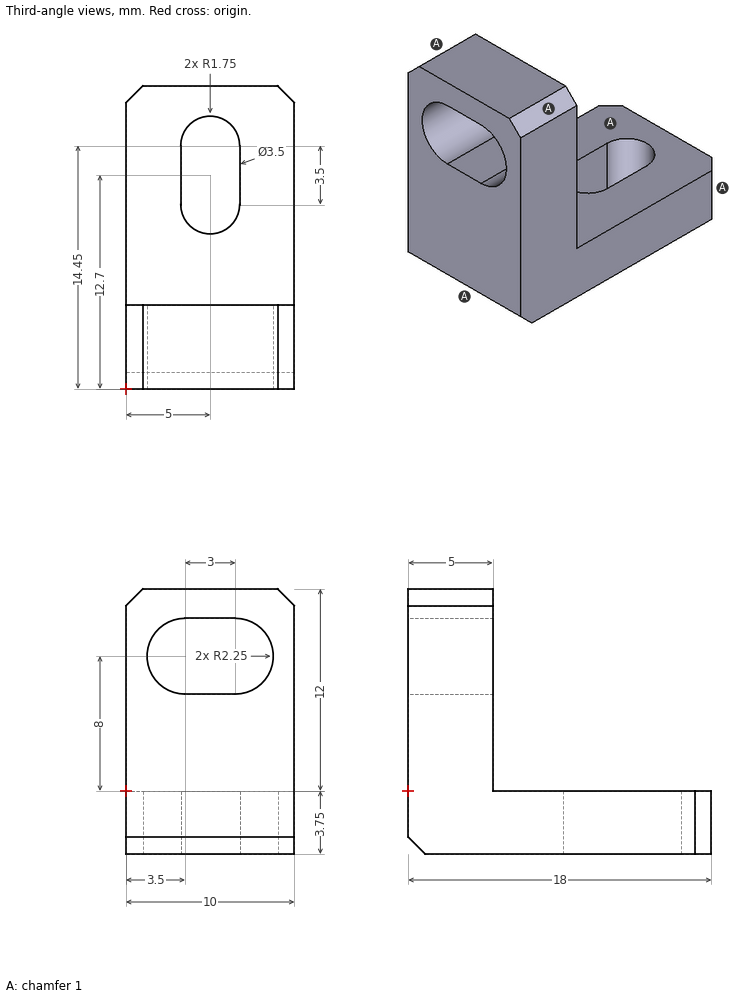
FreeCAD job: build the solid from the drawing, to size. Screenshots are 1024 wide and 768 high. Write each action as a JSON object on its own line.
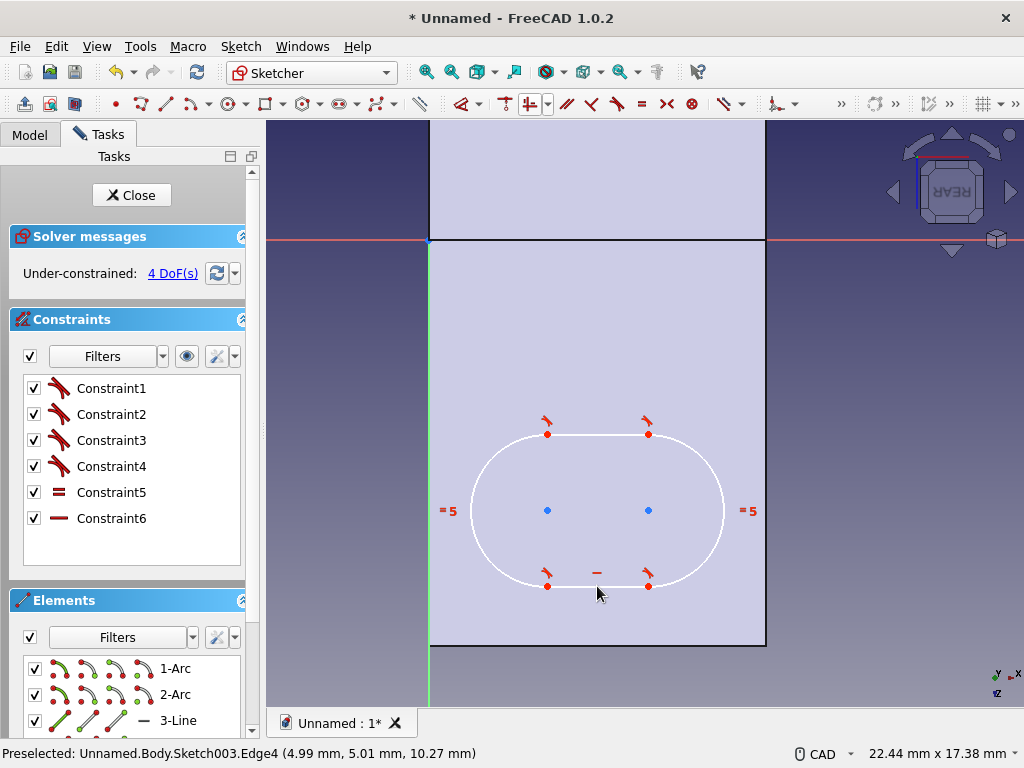
{"action": "left_click", "coordinate": [460, 104]}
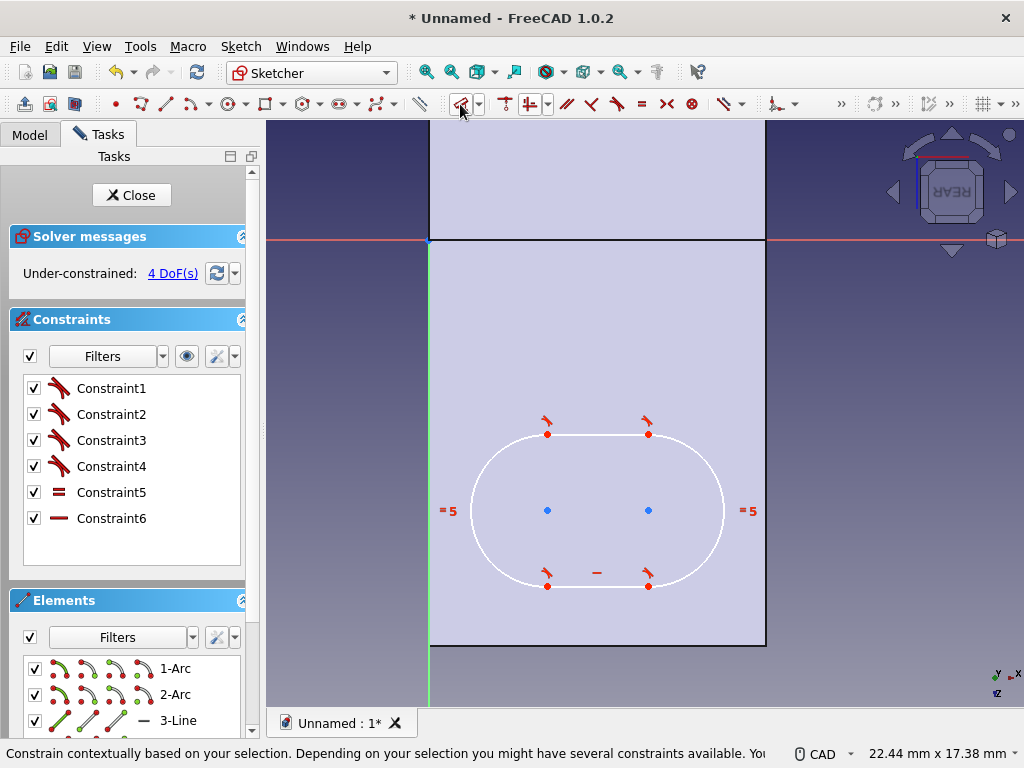
{"action": "left_click", "coordinate": [486, 466]}
{"action": "left_click", "coordinate": [460, 447]}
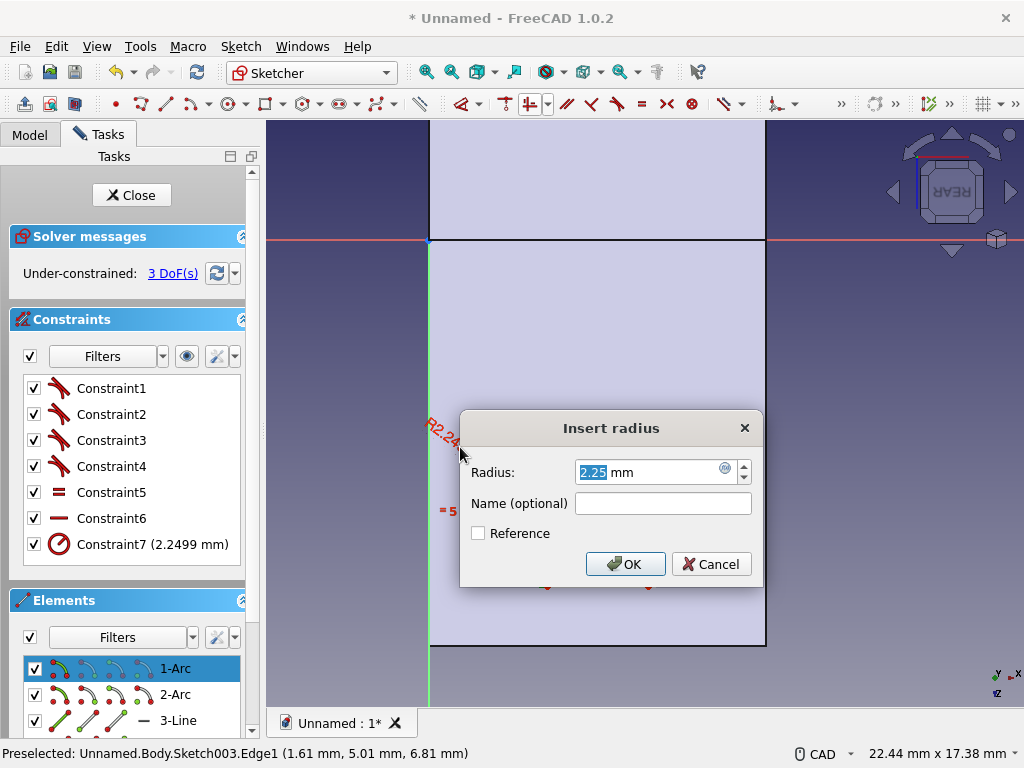
{"action": "type", "text": "2.25"}
{"action": "key", "text": "Return"}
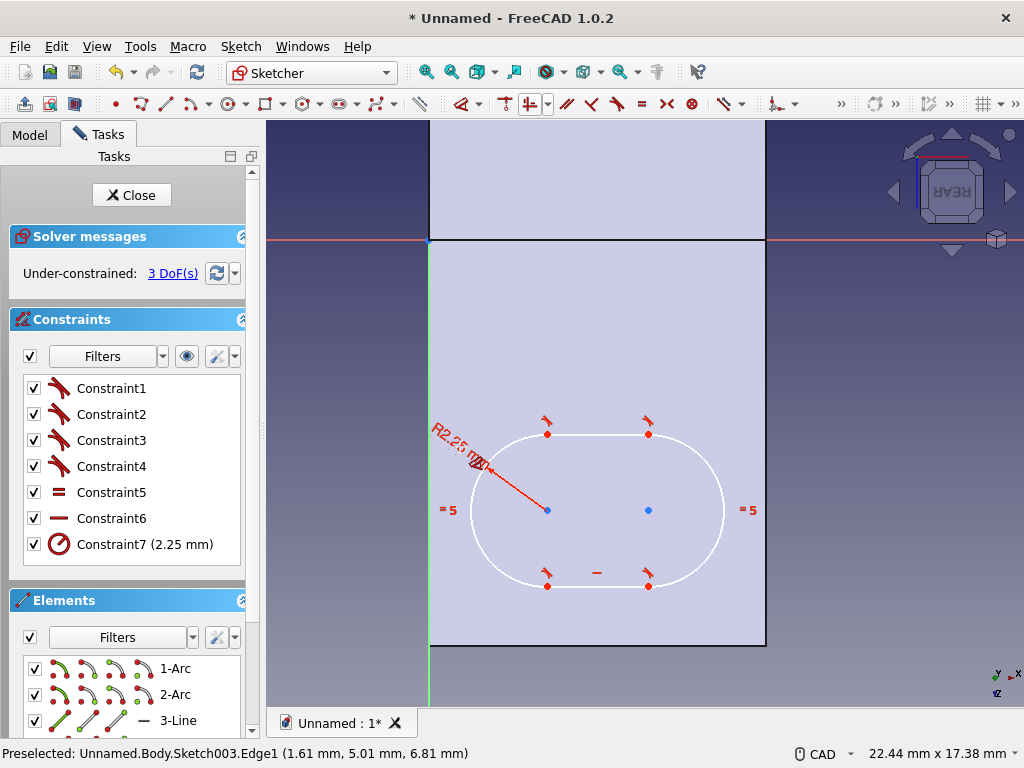
{"action": "left_click", "coordinate": [577, 435]}
{"action": "left_click", "coordinate": [598, 469]}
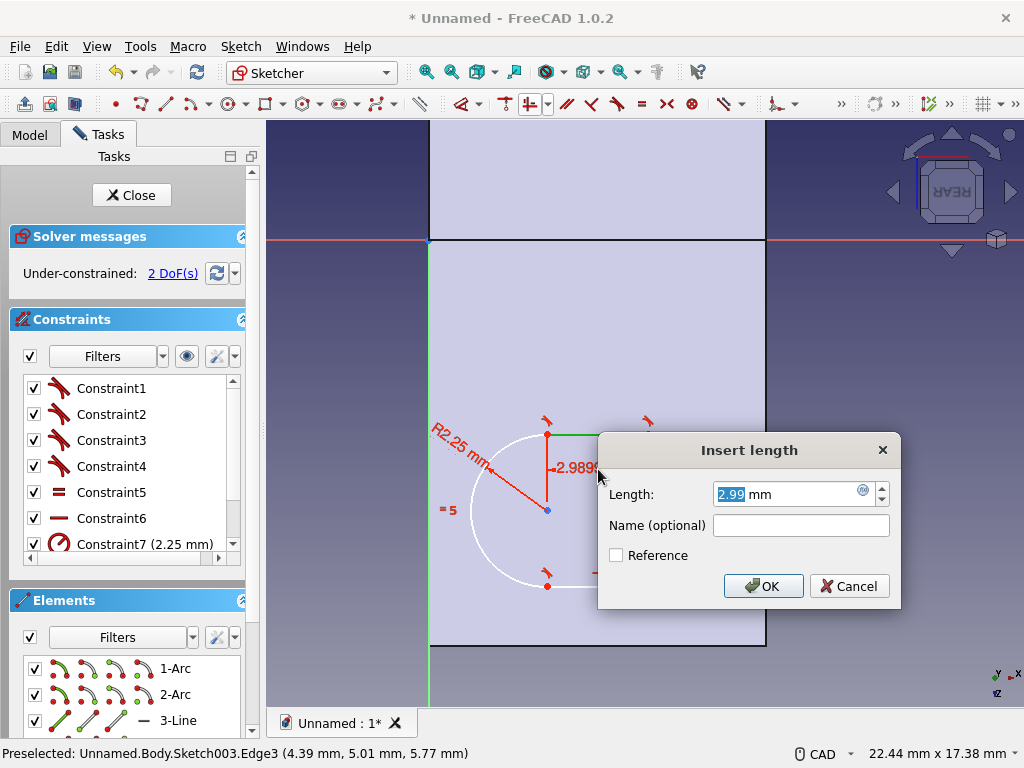
{"action": "type", "text": "3"}
{"action": "key", "text": "Return"}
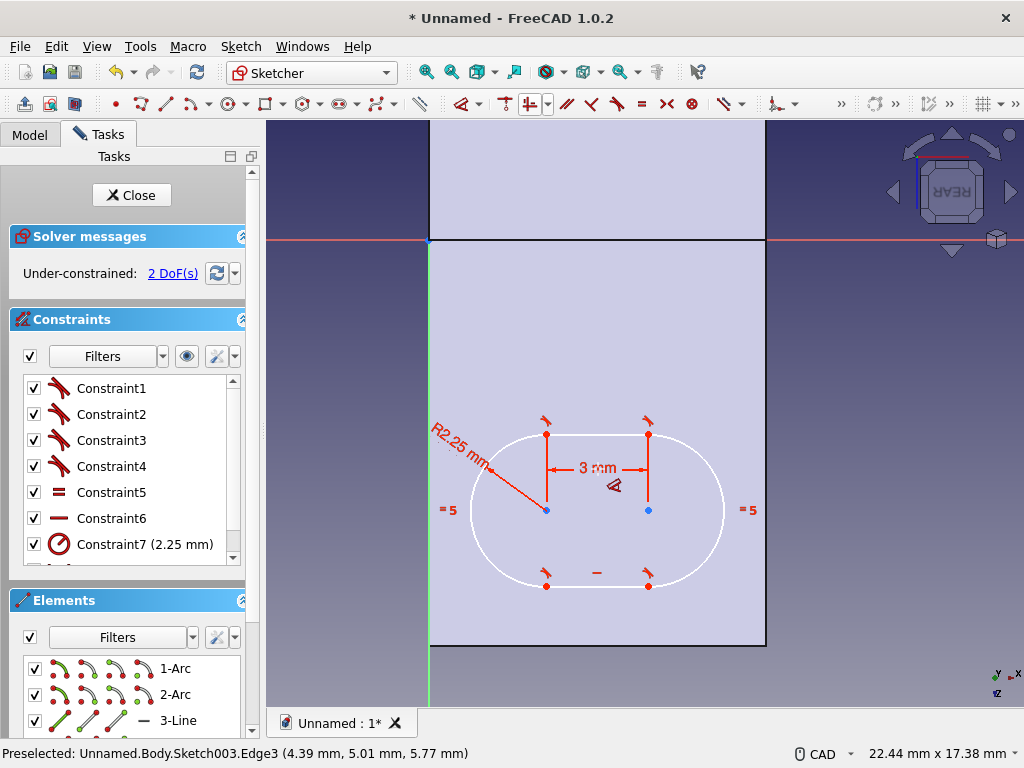
{"action": "left_click", "coordinate": [547, 511]}
{"action": "left_click", "coordinate": [395, 376]}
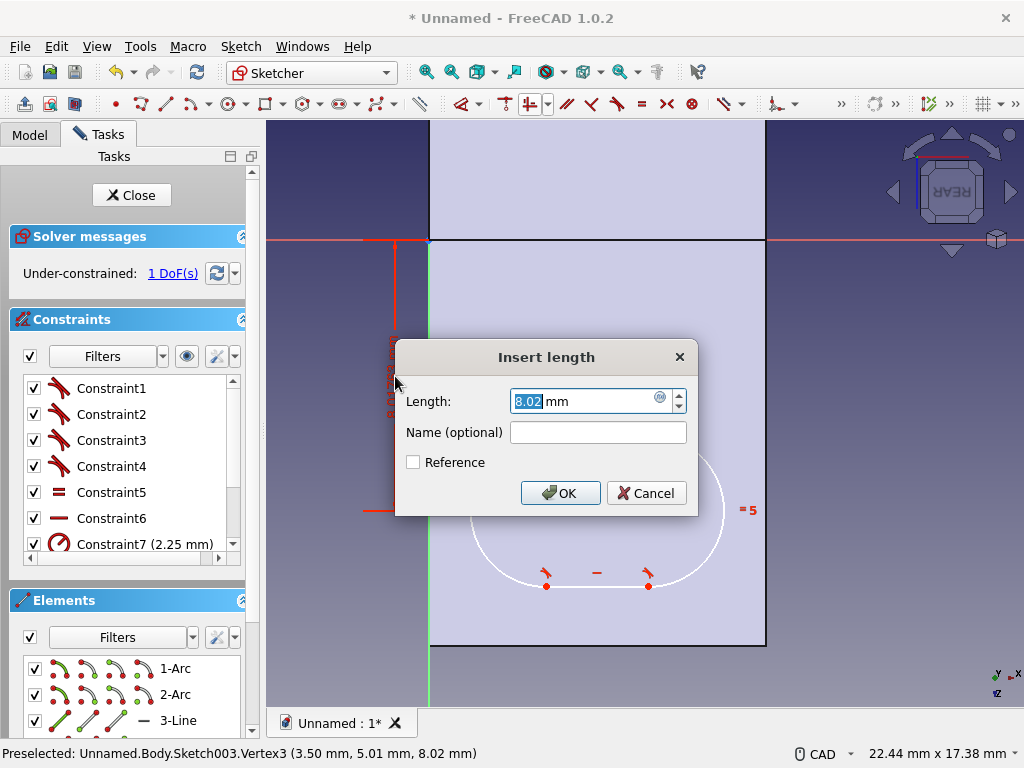
{"action": "type", "text": "8"}
{"action": "key", "text": "Return"}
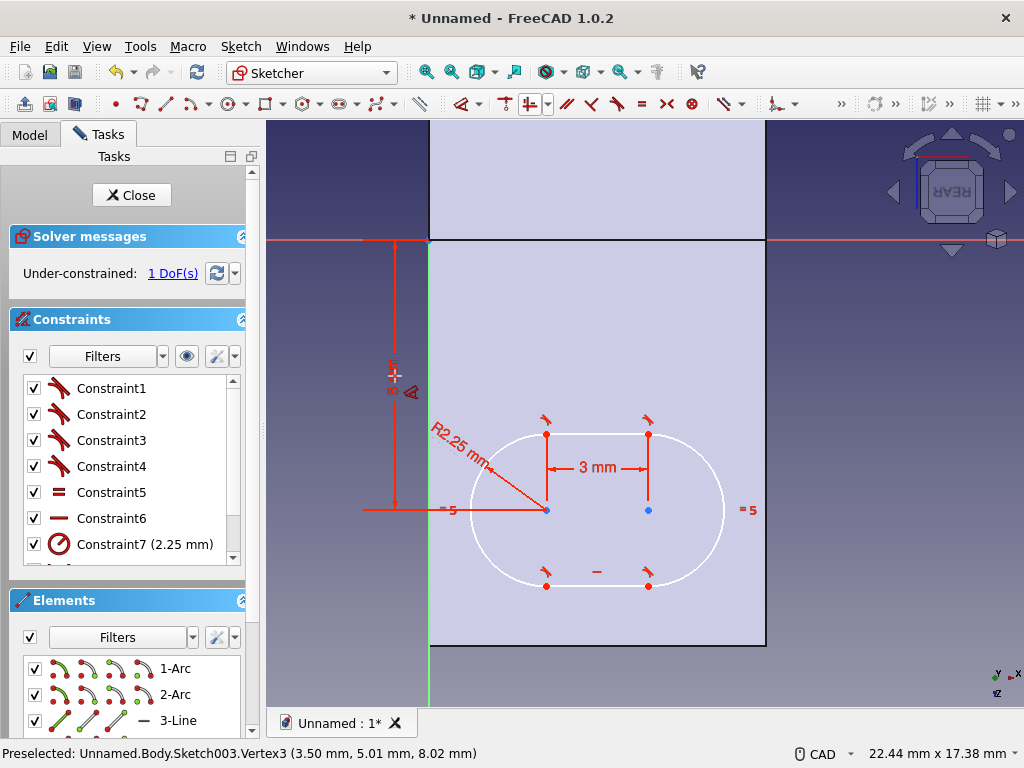
{"action": "left_click", "coordinate": [547, 434]}
{"action": "left_click", "coordinate": [488, 206]}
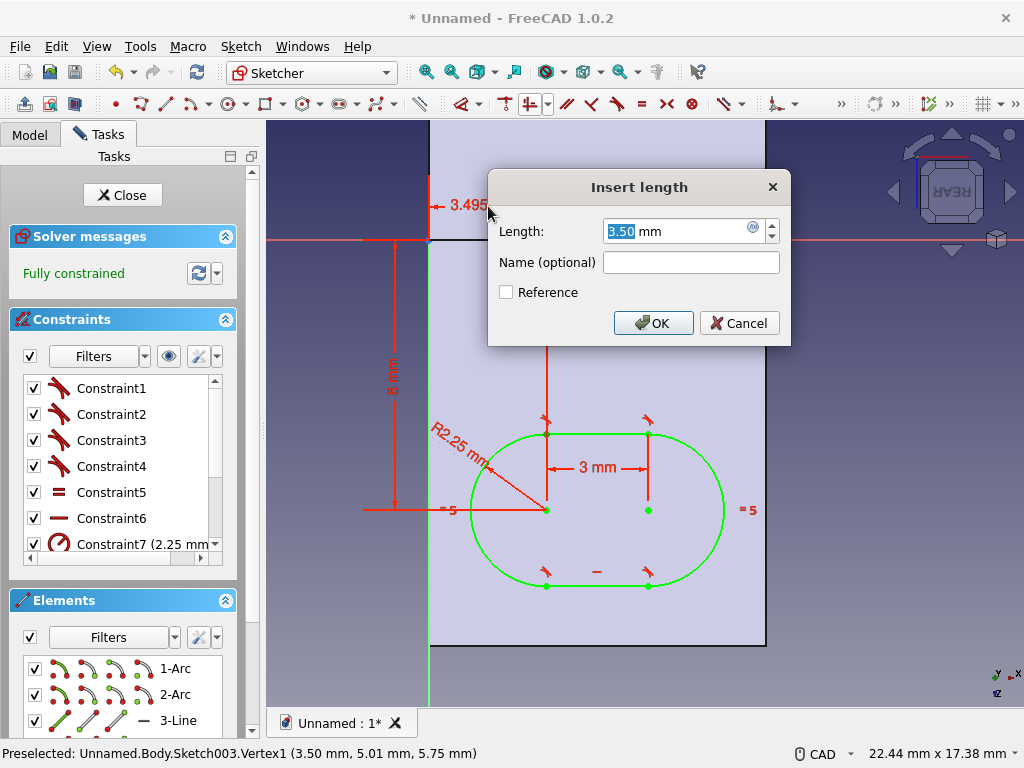
{"action": "type", "text": "3.5"}
{"action": "key", "text": "Return"}
{"action": "key", "text": "Escape"}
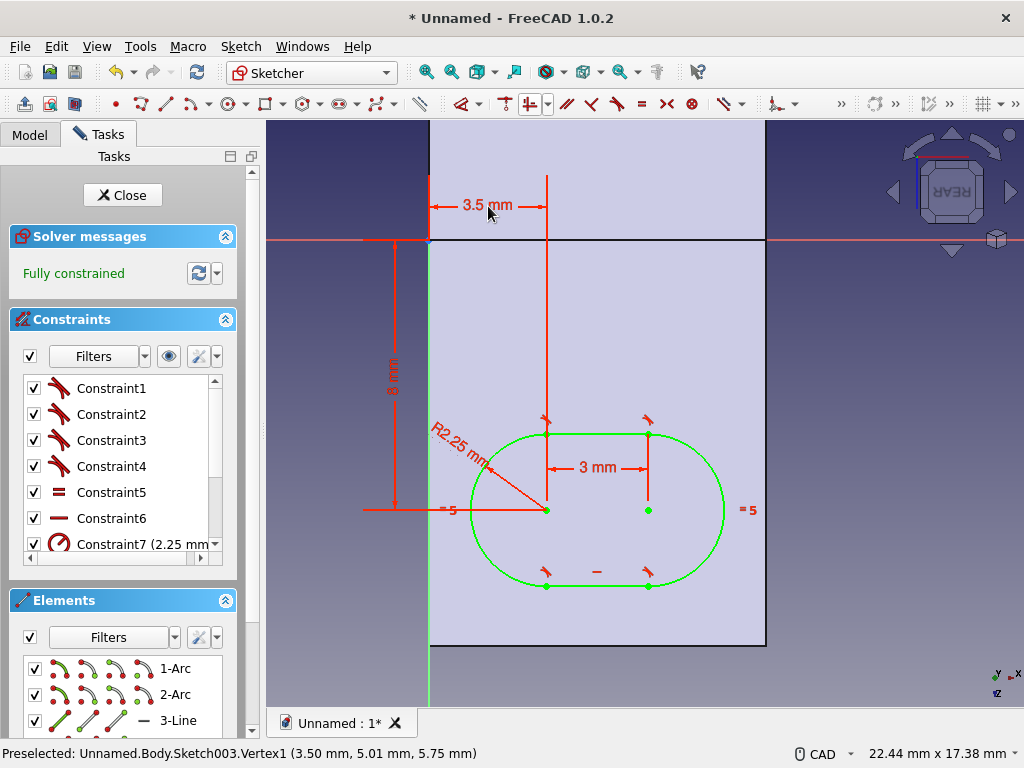
{"action": "left_click", "coordinate": [123, 195]}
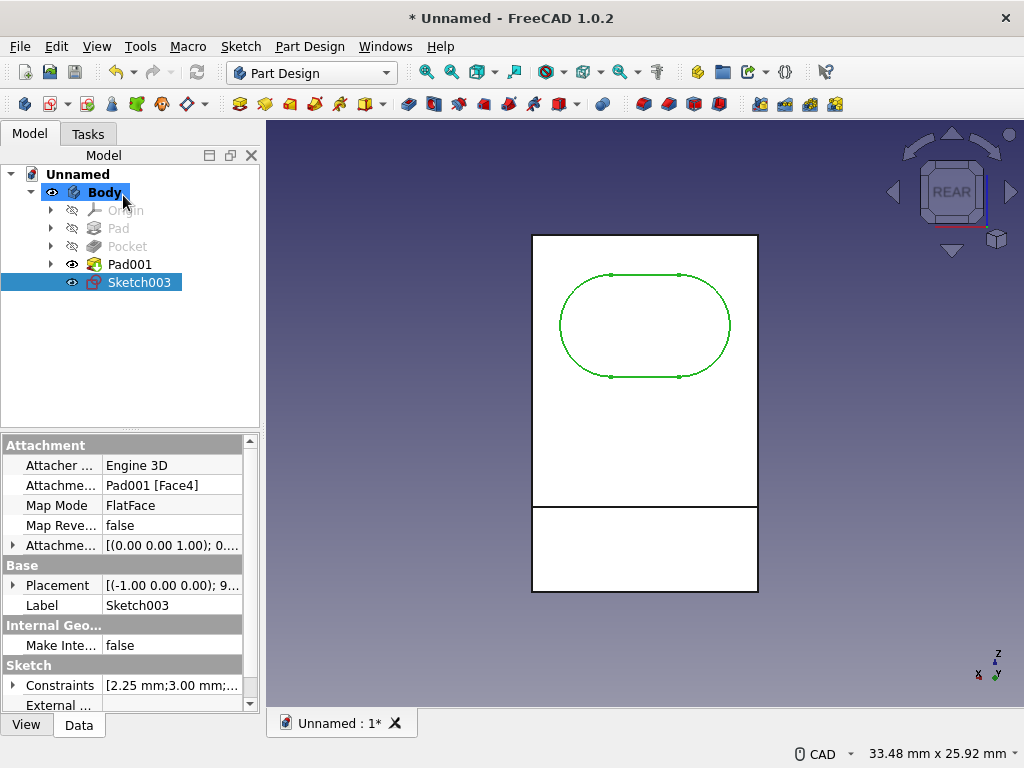
{"action": "left_click", "coordinate": [409, 104]}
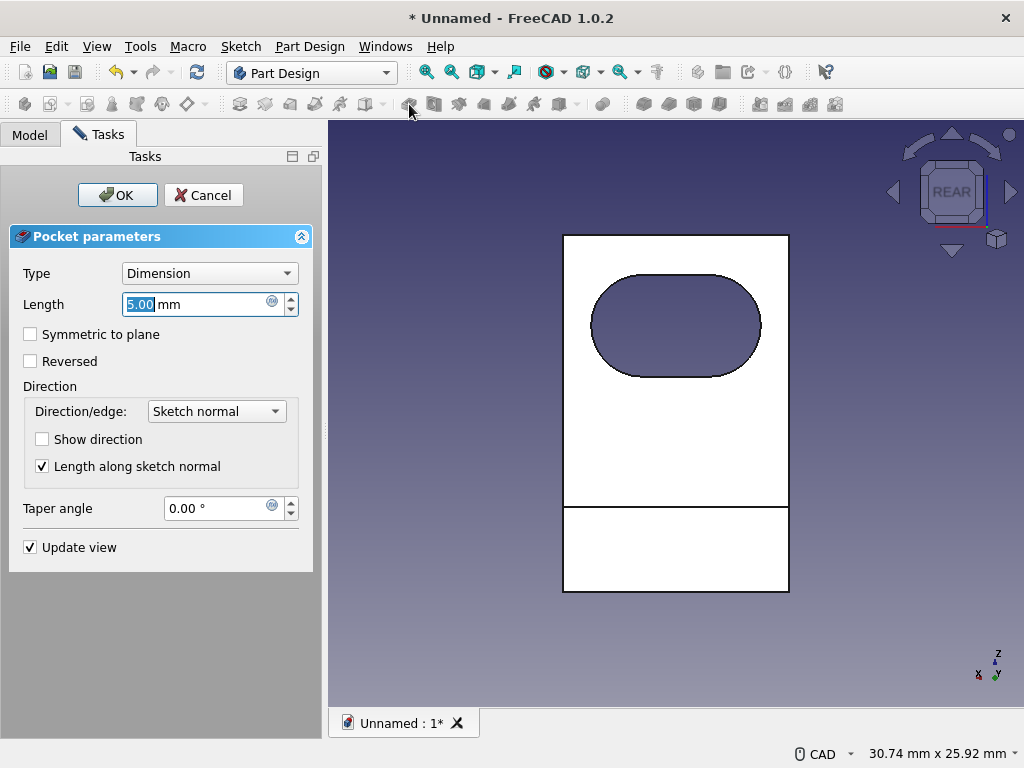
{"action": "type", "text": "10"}
{"action": "key", "text": "Tab"}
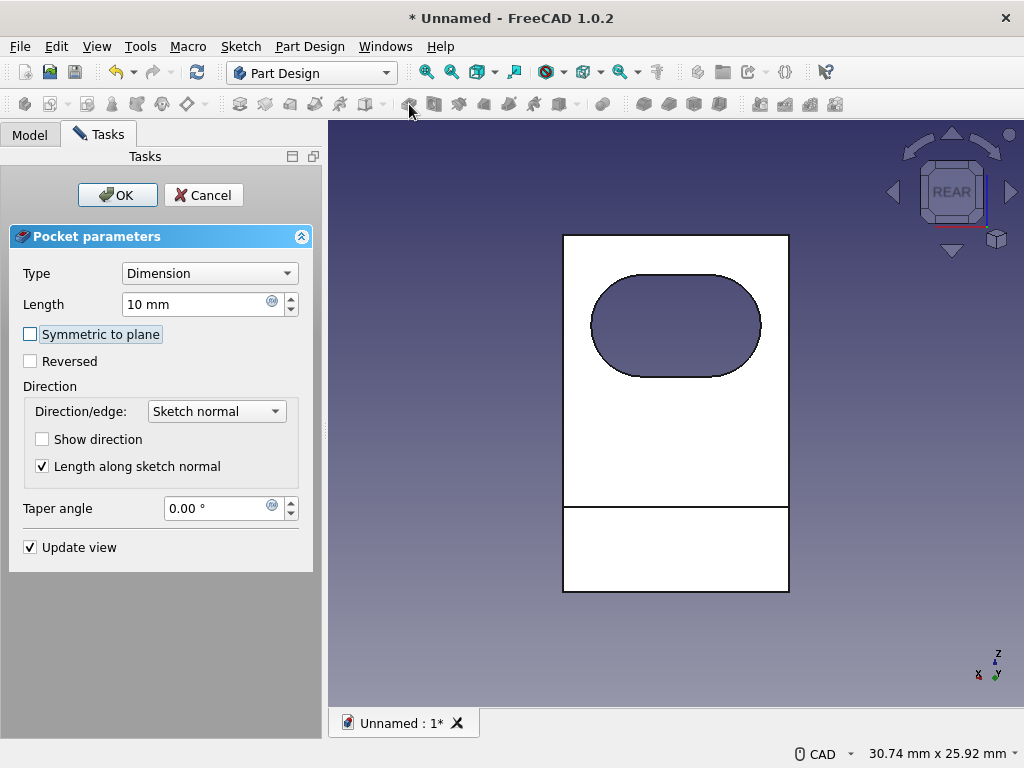
{"action": "left_click", "coordinate": [118, 195]}